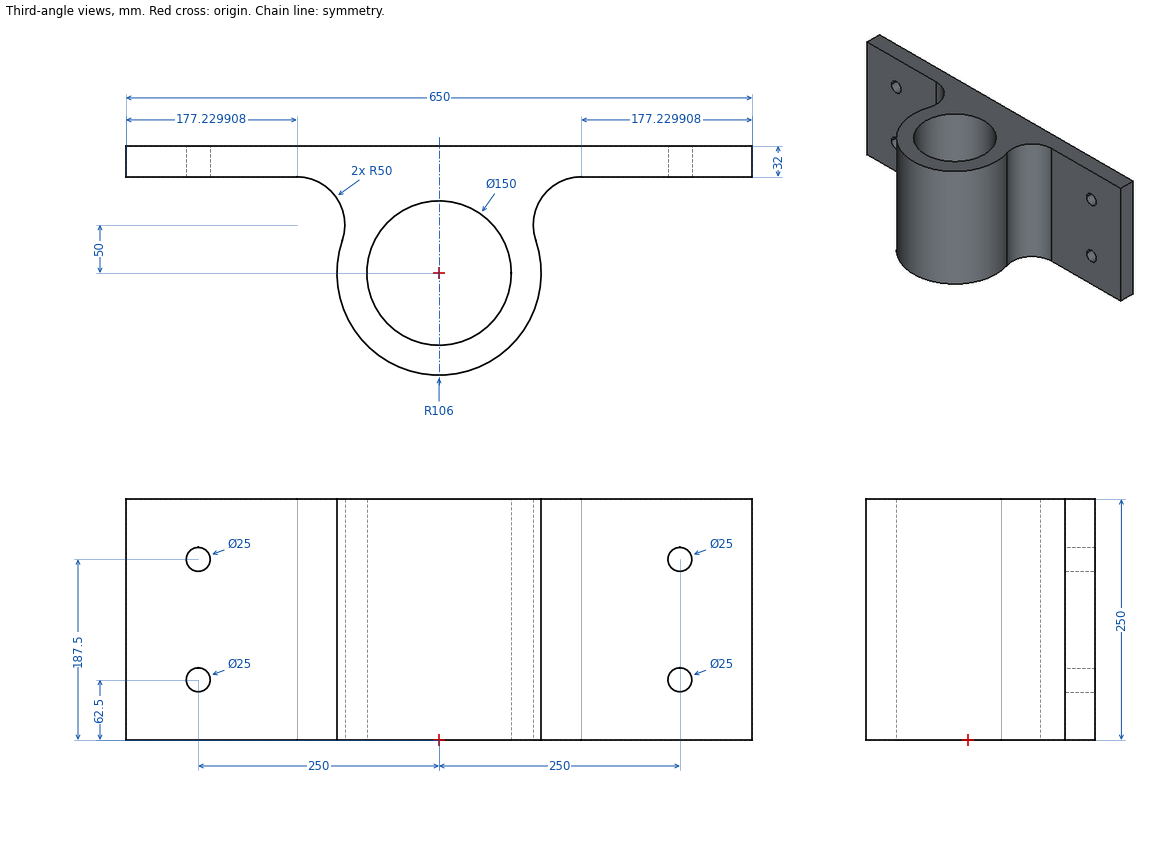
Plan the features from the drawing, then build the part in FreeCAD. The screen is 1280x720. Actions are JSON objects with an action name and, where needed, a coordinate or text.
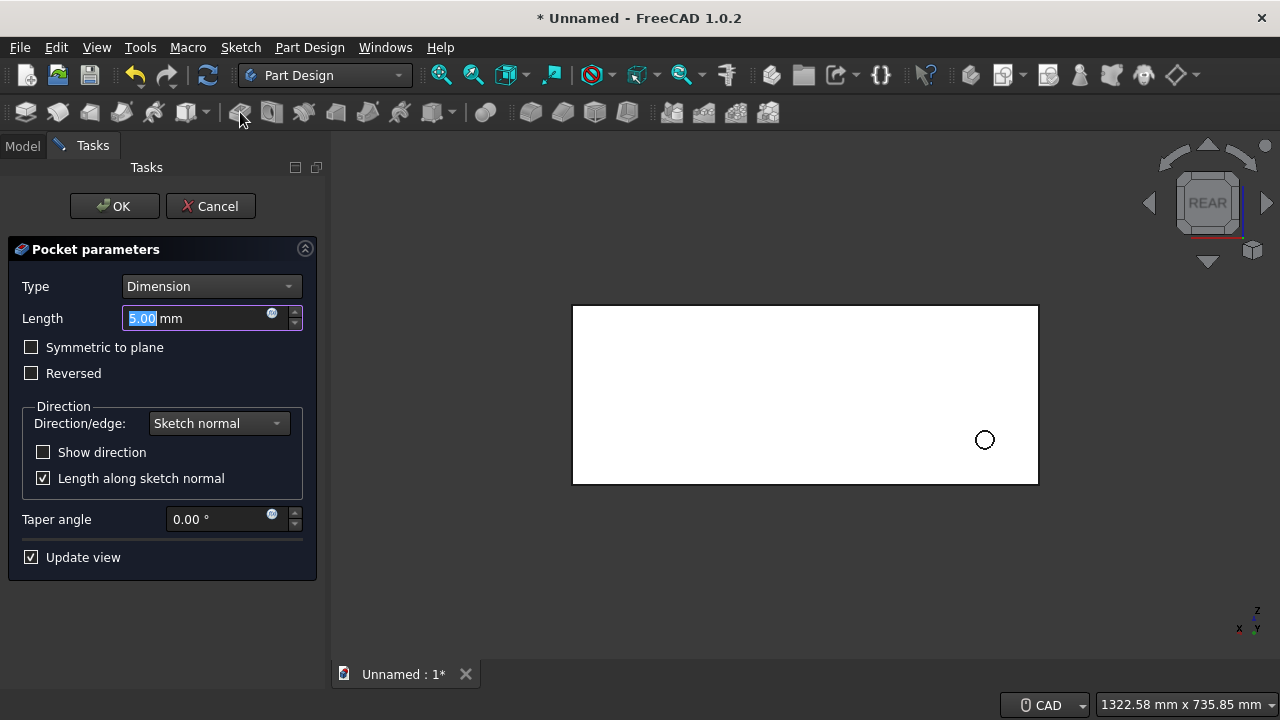
{"action": "left_click", "coordinate": [212, 286]}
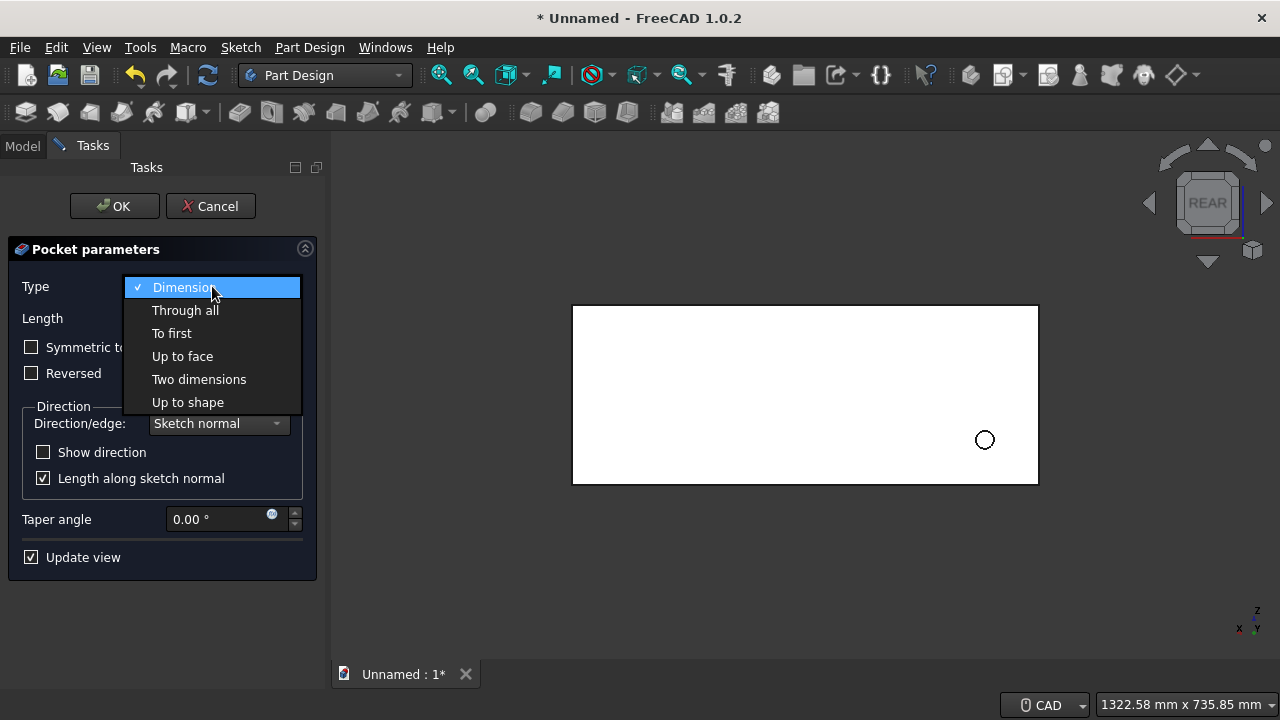
{"action": "left_click", "coordinate": [212, 334]}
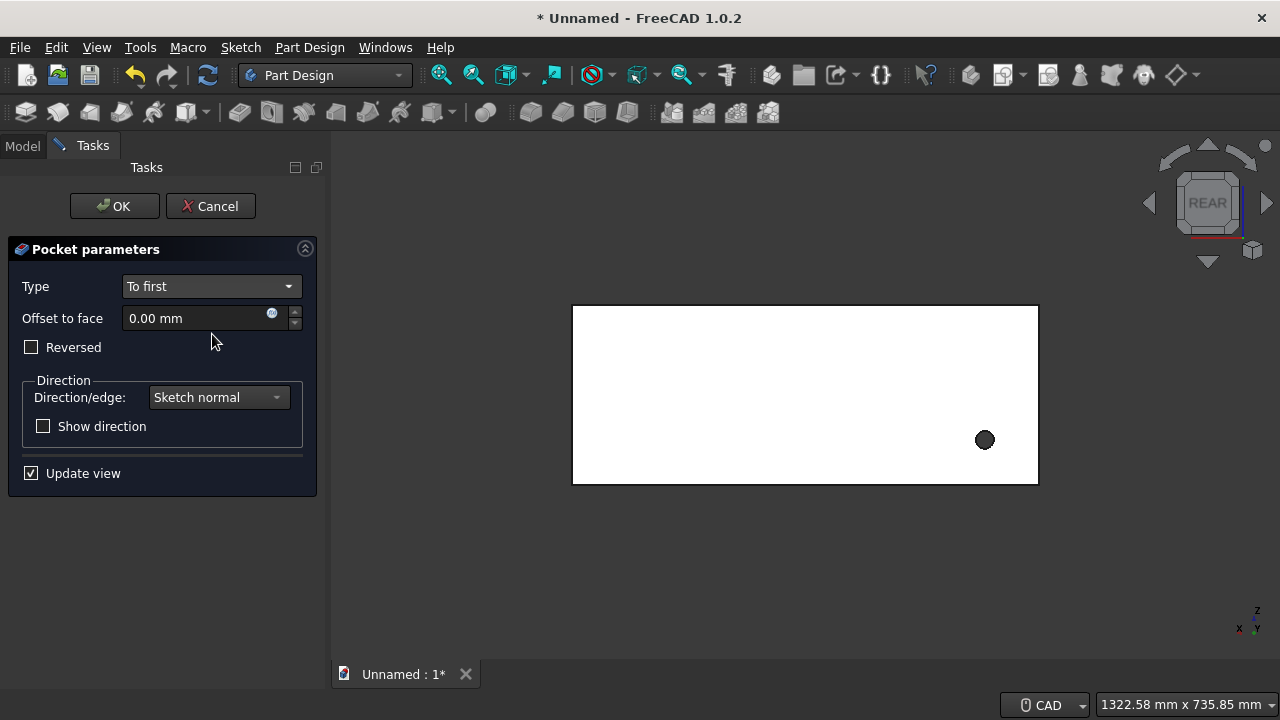
{"action": "left_click", "coordinate": [115, 206]}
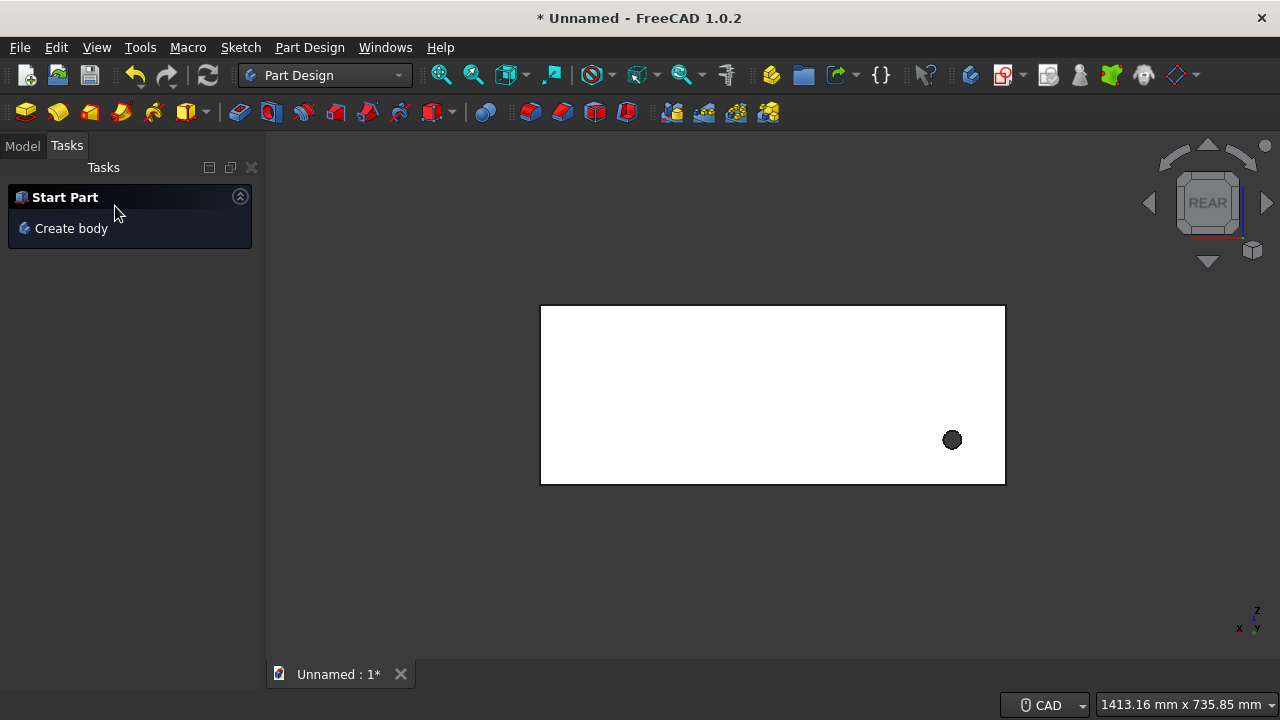
{"action": "left_click", "coordinate": [640, 394]}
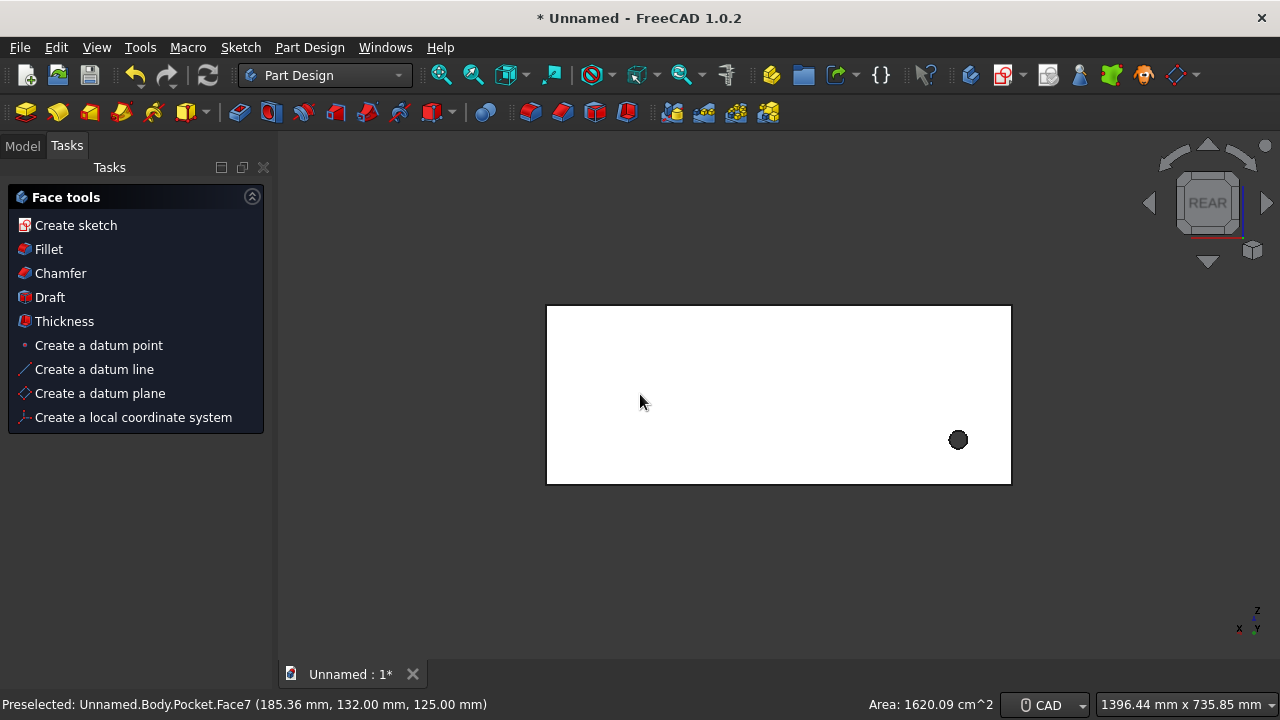
{"action": "left_click", "coordinate": [1004, 76]}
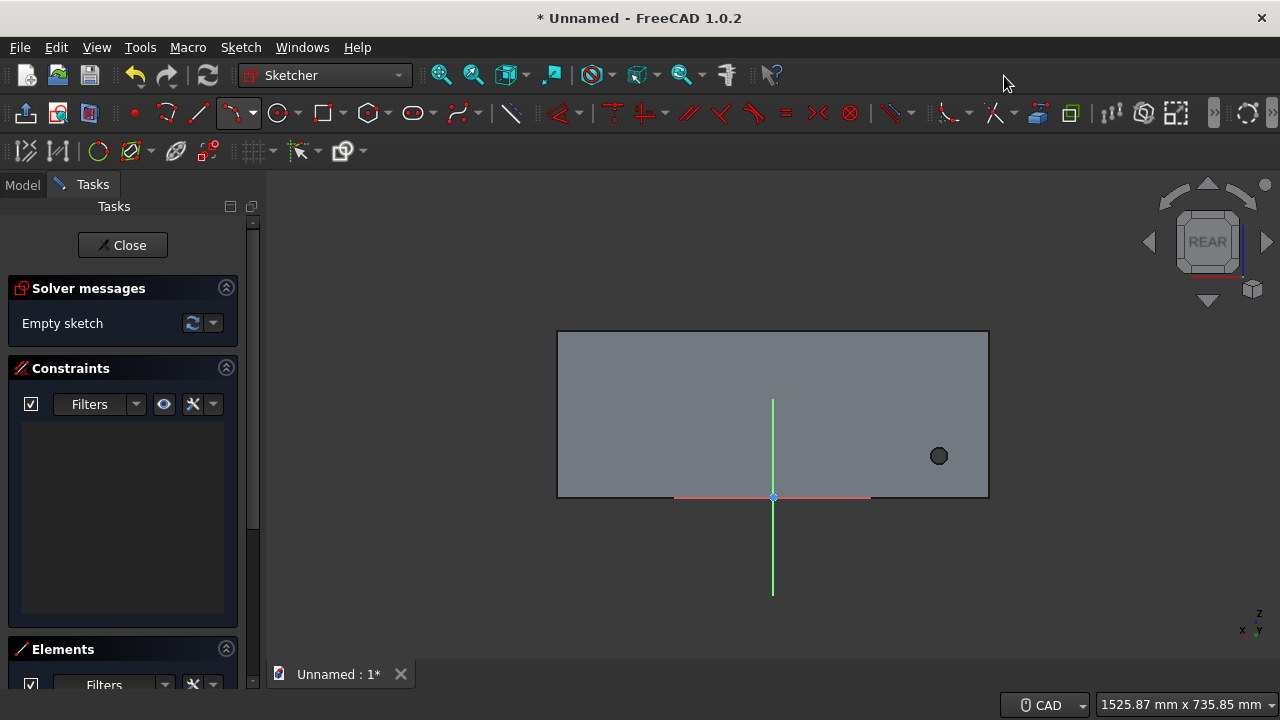
{"action": "scroll", "coordinate": [951, 371], "scroll_direction": "up", "scroll_amount": 15}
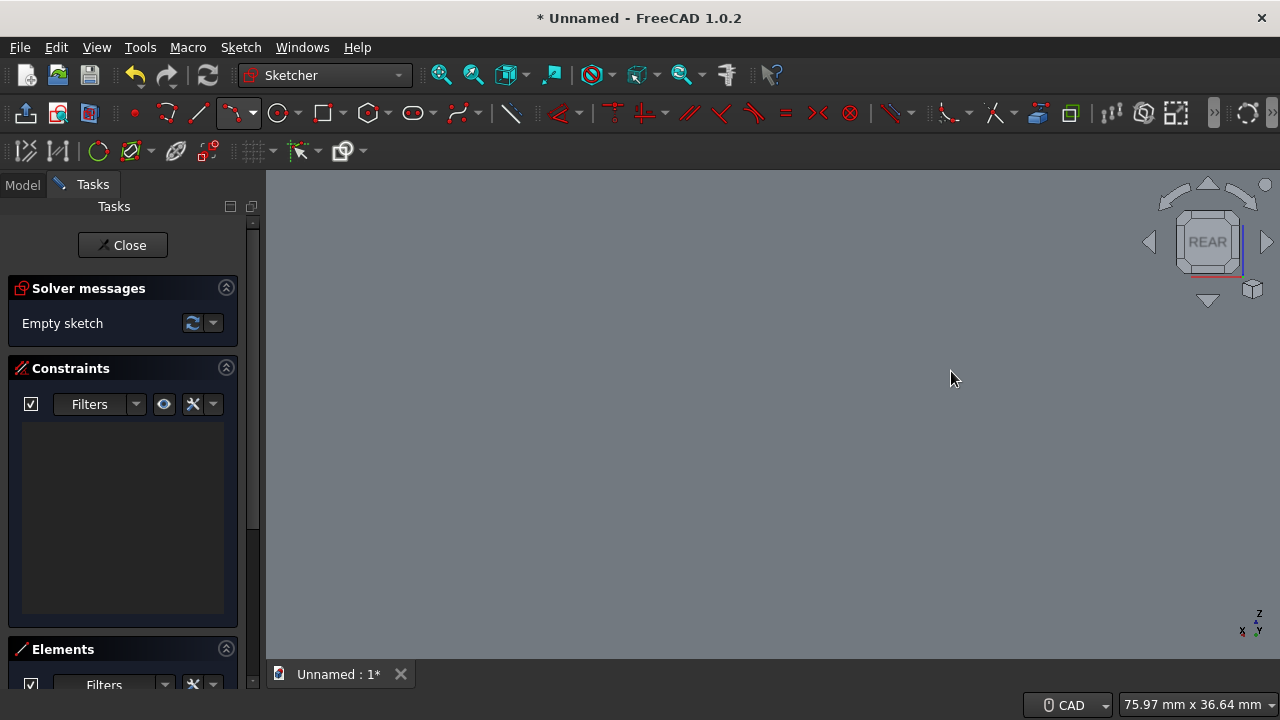
{"action": "left_click", "coordinate": [278, 114]}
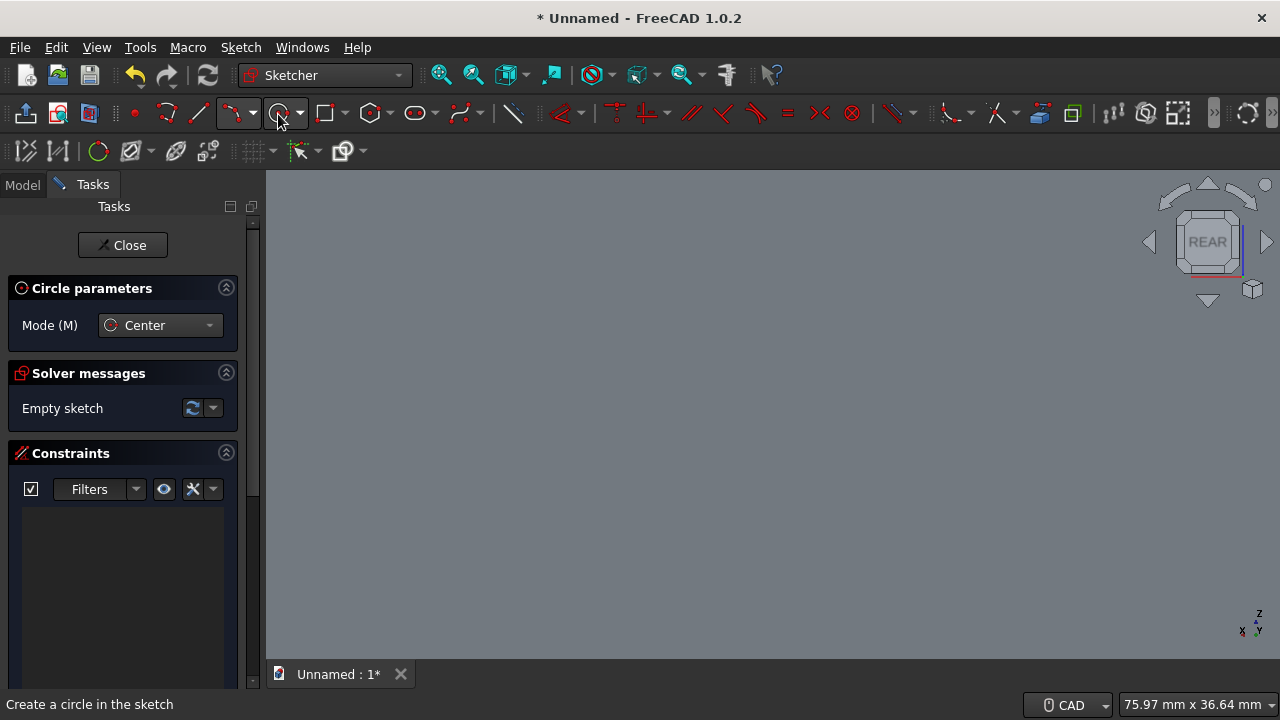
{"action": "left_click", "coordinate": [700, 403]}
{"action": "mouse_move", "coordinate": [818, 285]}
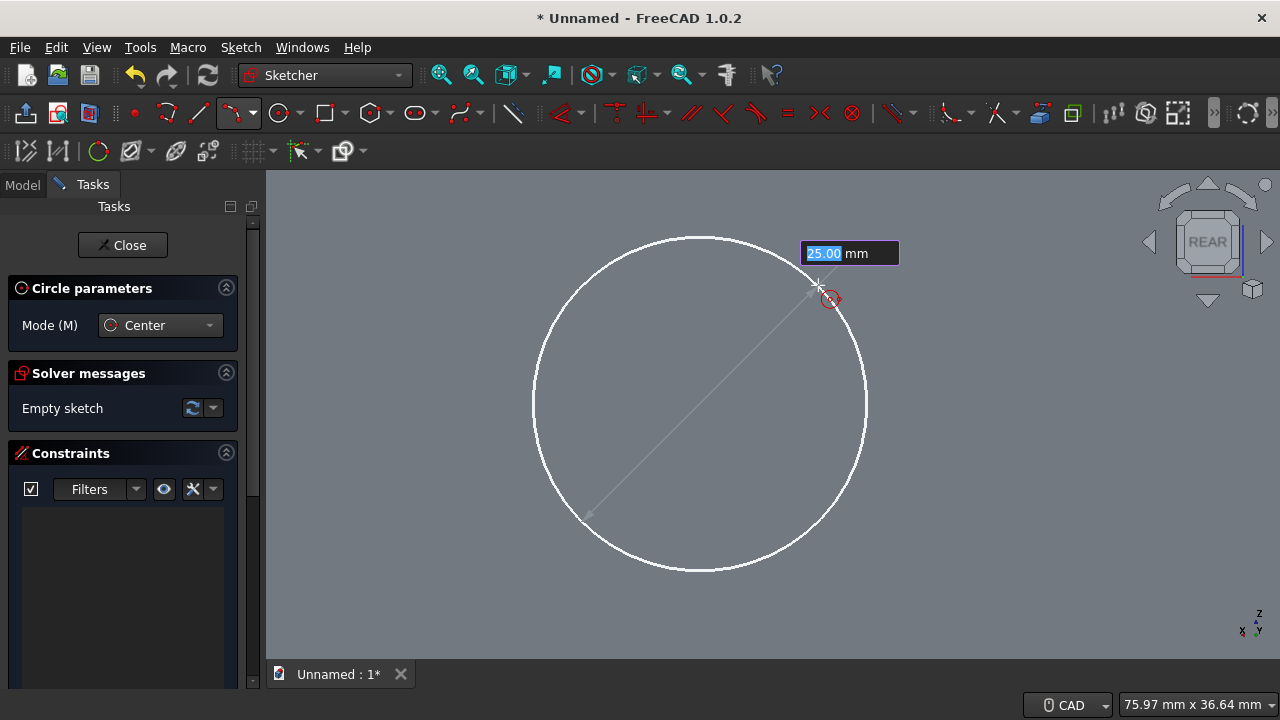
{"action": "type", "text": "25"}
{"action": "key", "text": "Return"}
{"action": "key", "text": "Escape"}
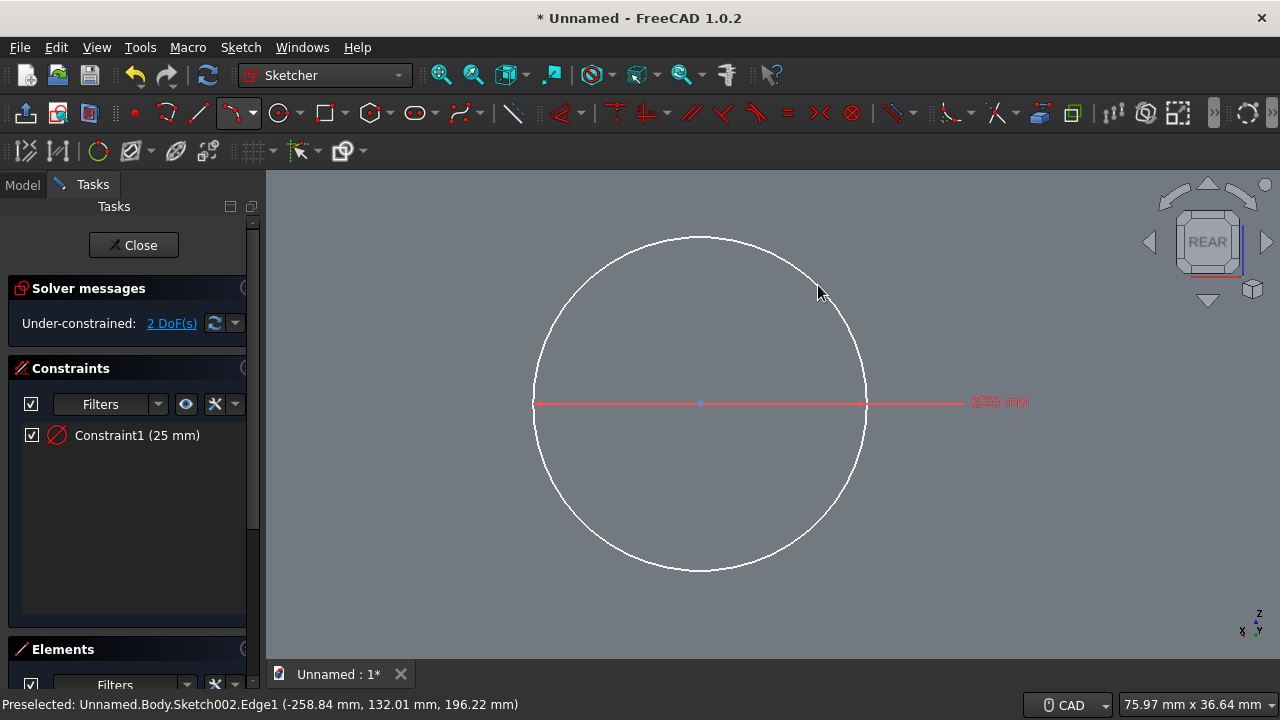
{"action": "left_click", "coordinate": [560, 114]}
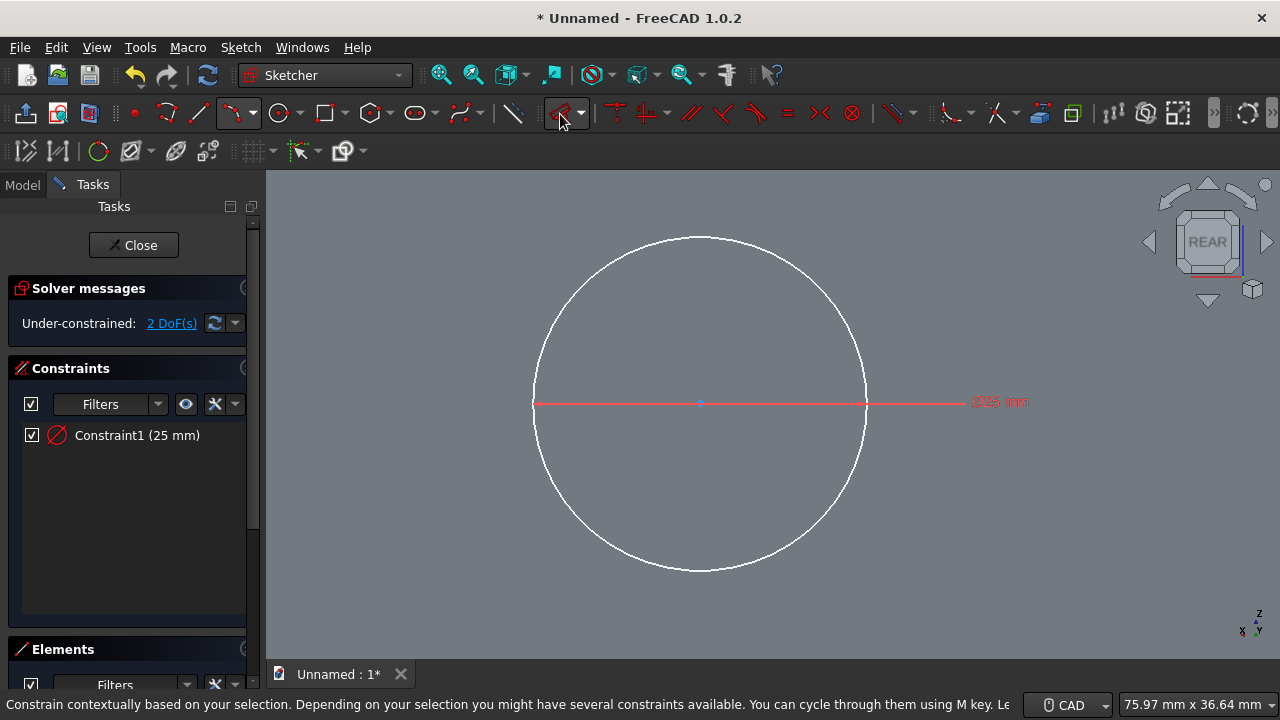
{"action": "left_click", "coordinate": [700, 404]}
{"action": "left_click", "coordinate": [497, 370]}